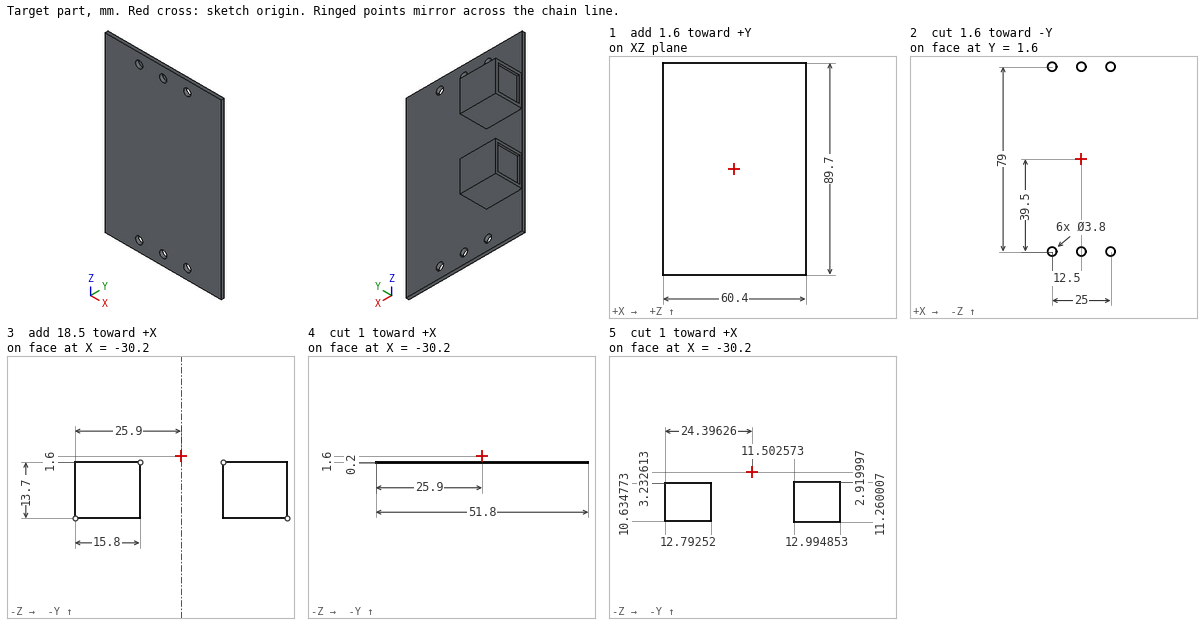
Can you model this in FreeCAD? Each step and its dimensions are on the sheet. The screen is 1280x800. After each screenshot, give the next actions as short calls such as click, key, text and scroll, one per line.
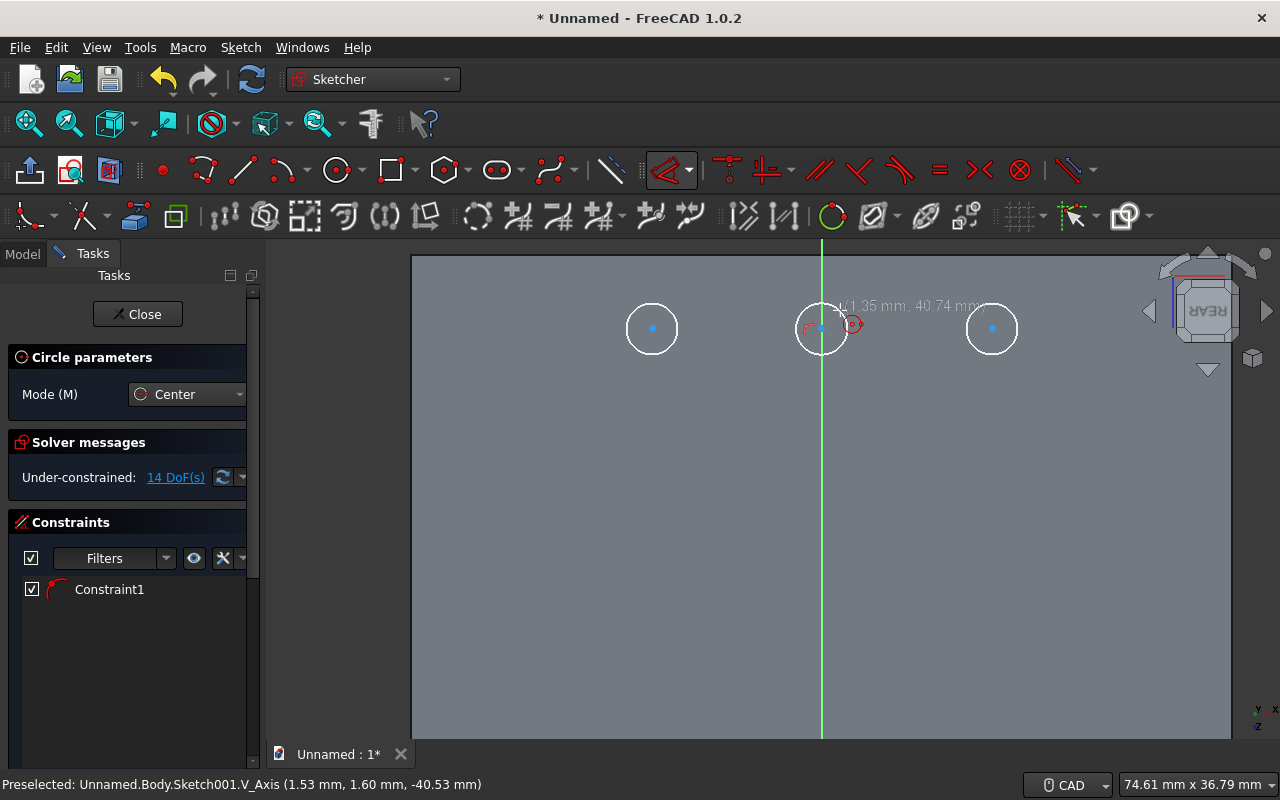
scroll(654, 327, down, 6)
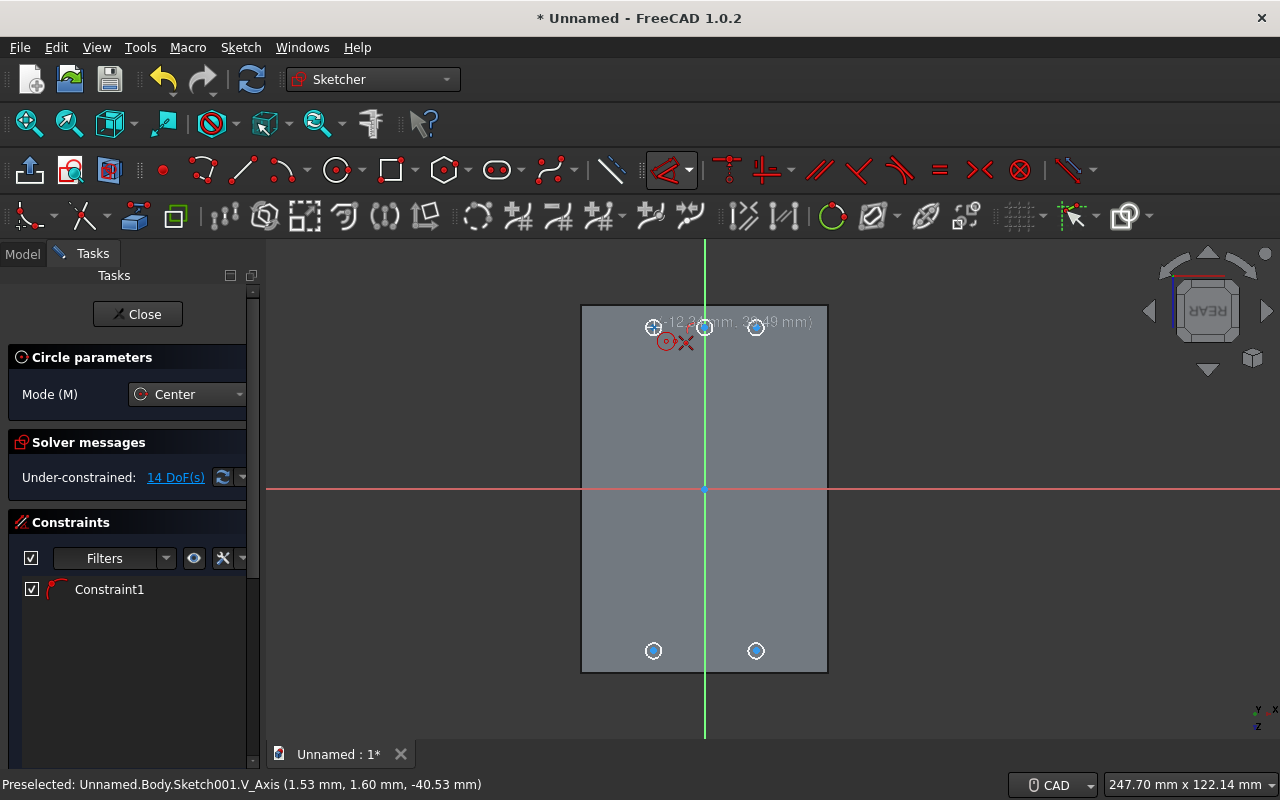
scroll(705, 651, up, 6)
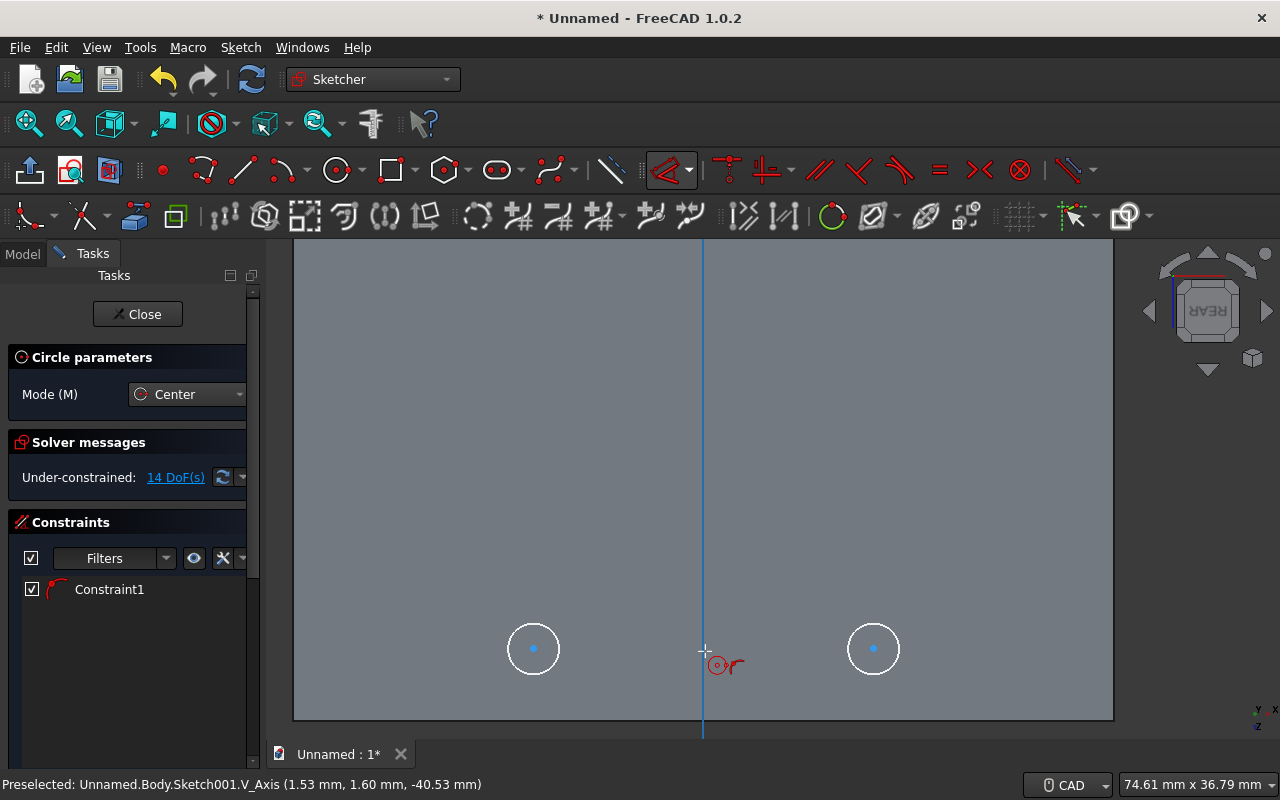
click(703, 648)
click(722, 630)
key(Escape)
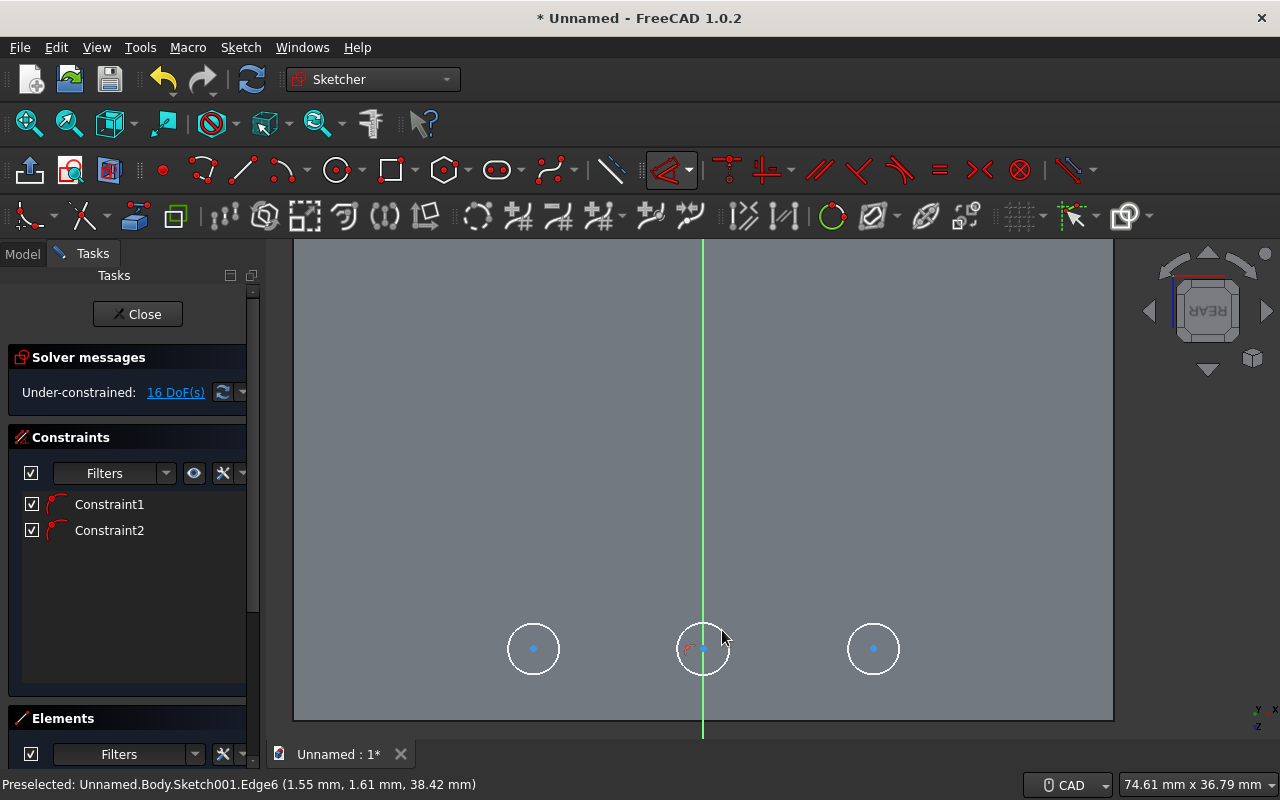
click(552, 631)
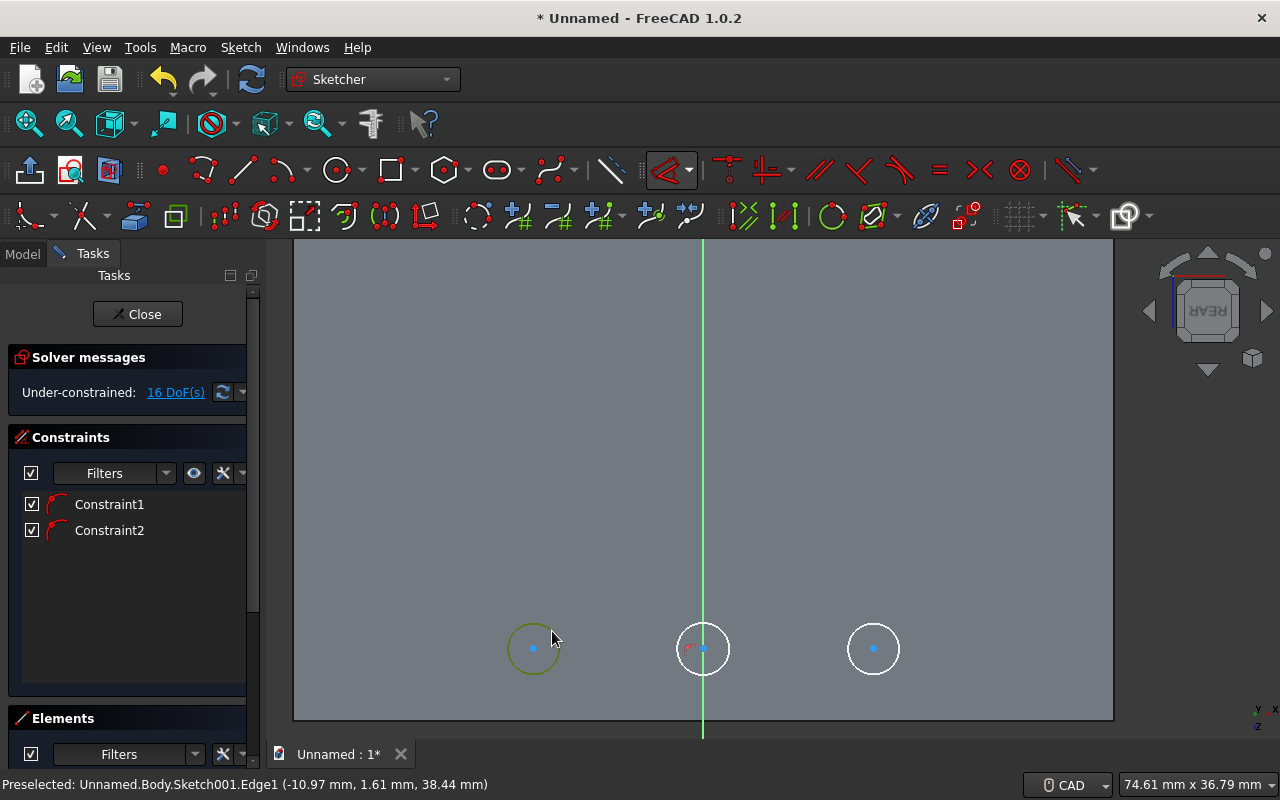
click(892, 631)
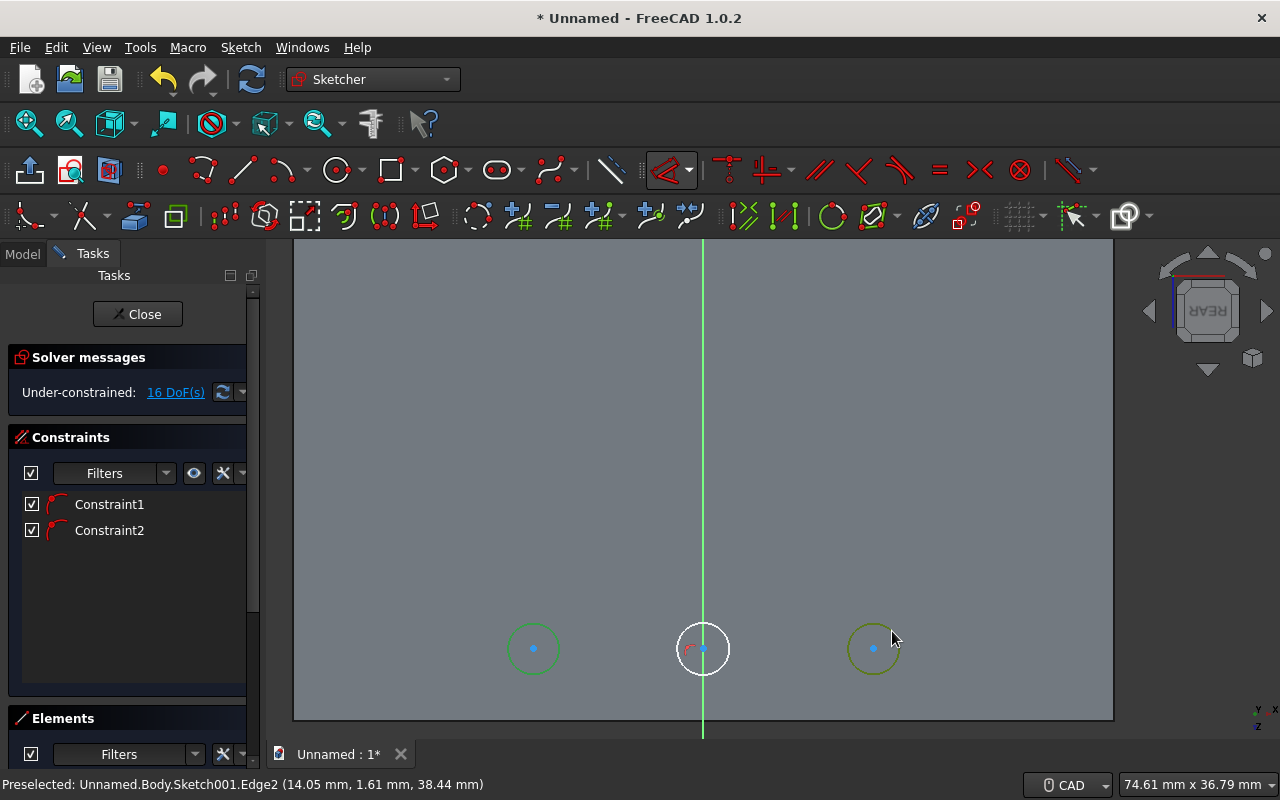
scroll(705, 652, down, 6)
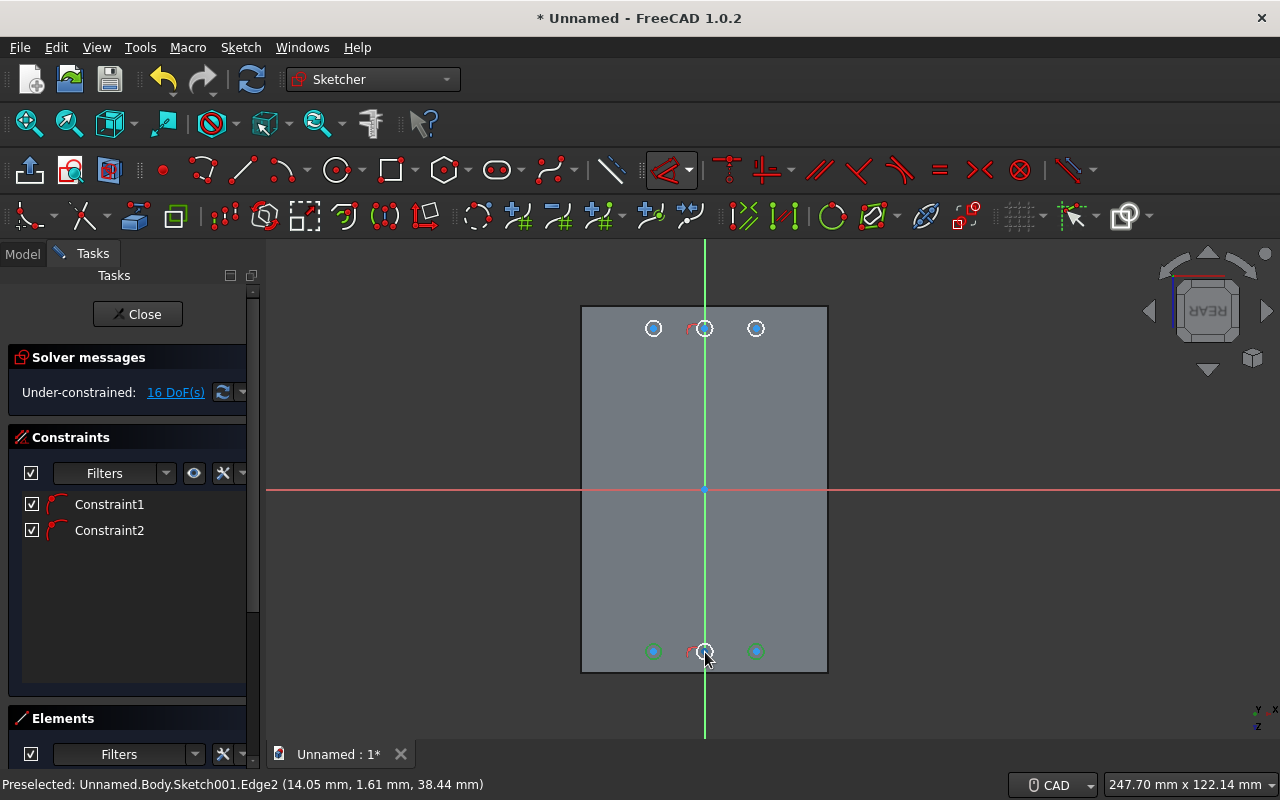
scroll(659, 323, up, 3)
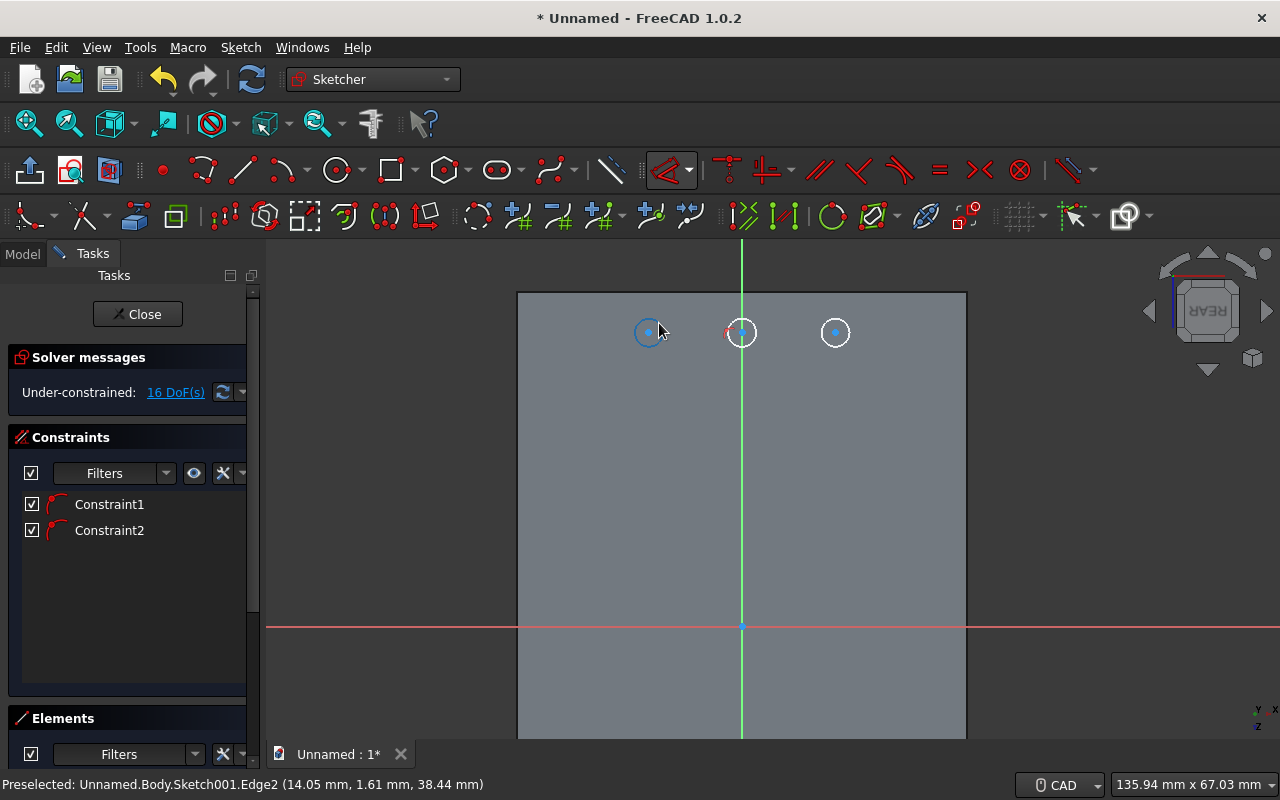
click(659, 323)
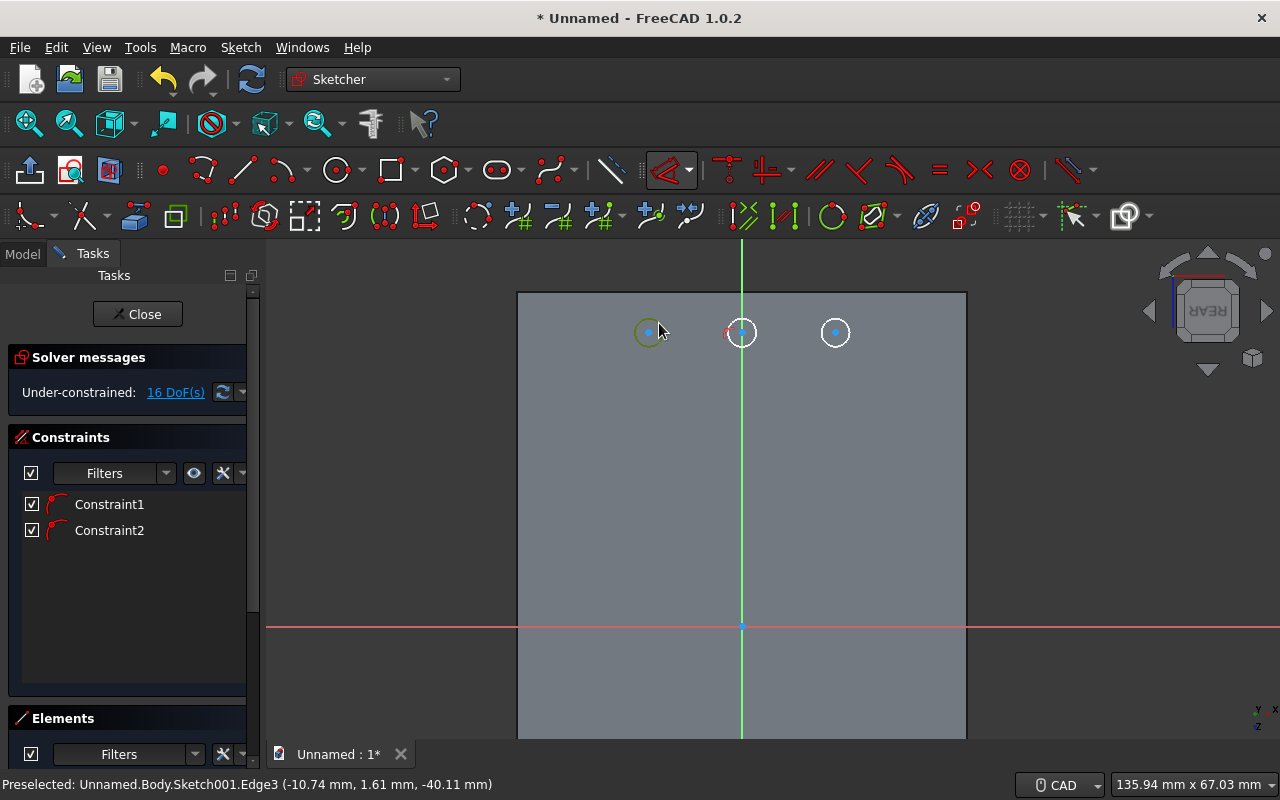
click(845, 323)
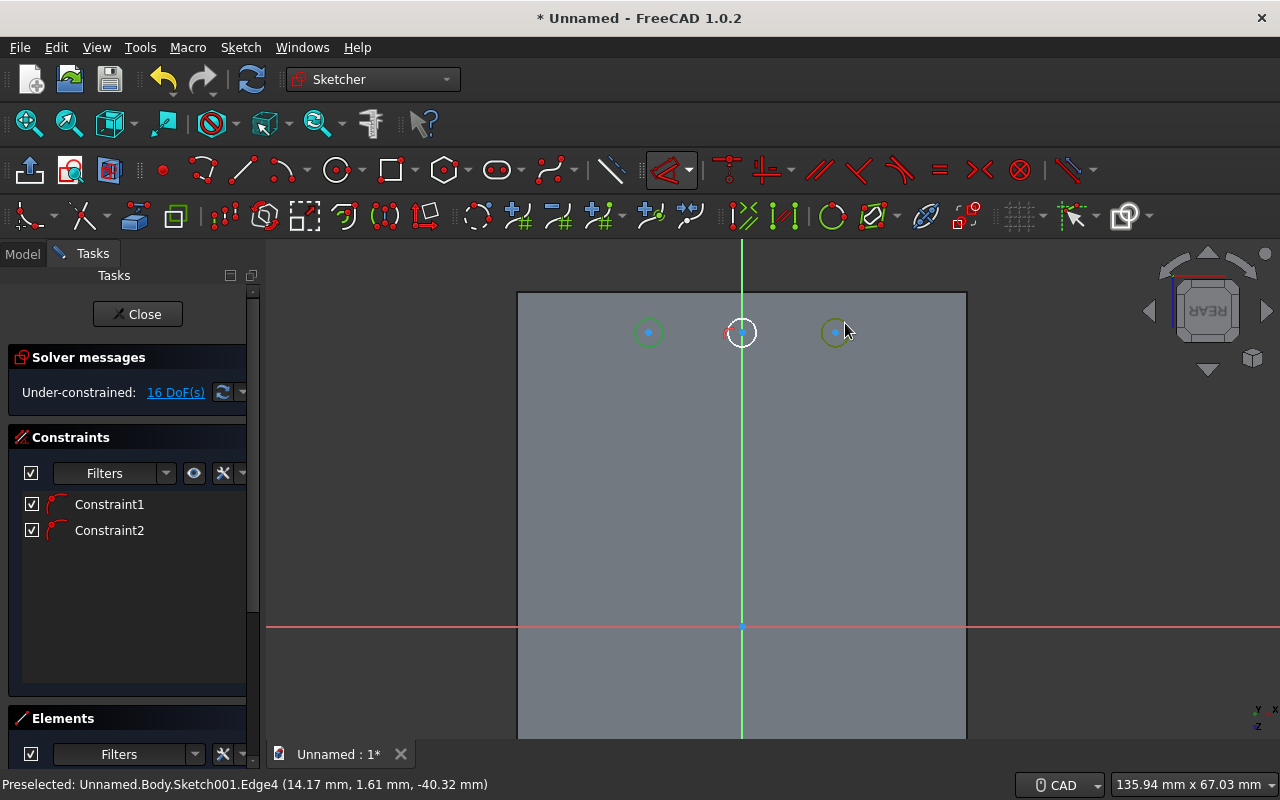
scroll(752, 323, up, 2)